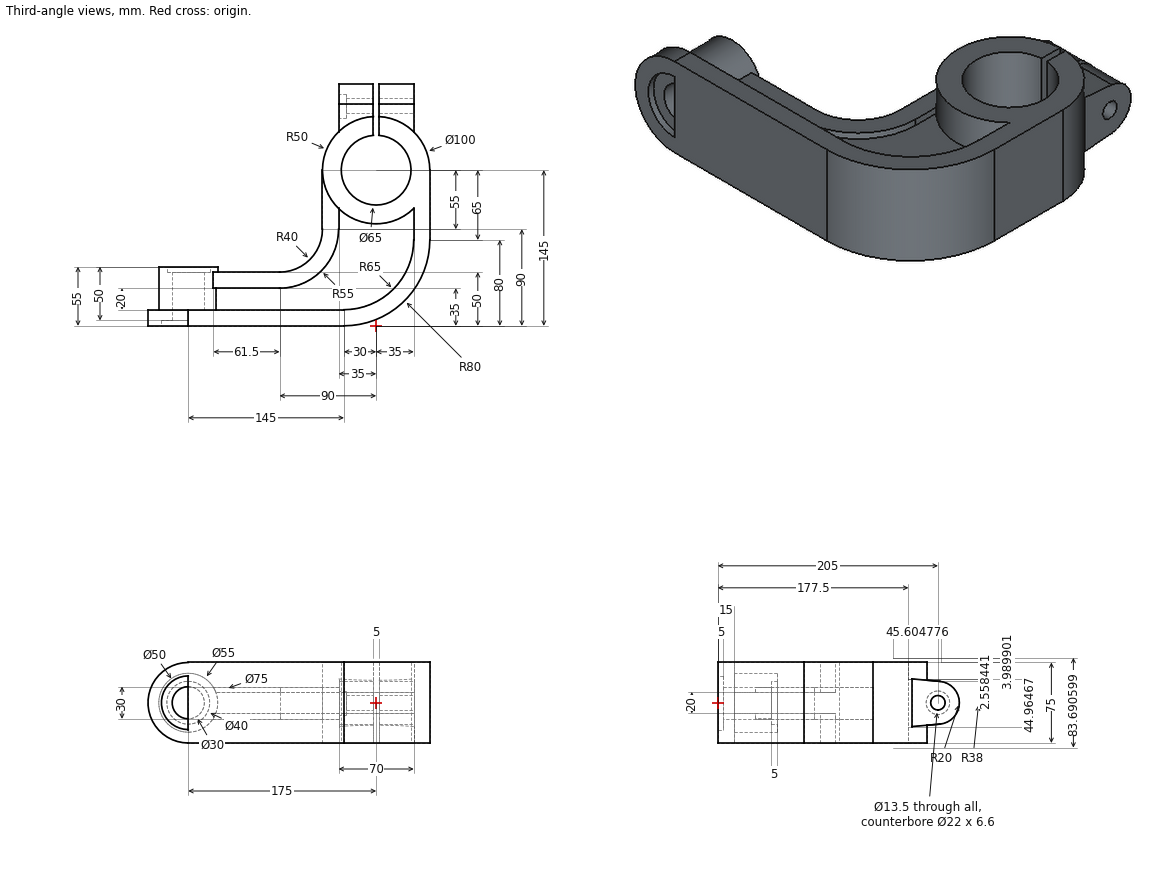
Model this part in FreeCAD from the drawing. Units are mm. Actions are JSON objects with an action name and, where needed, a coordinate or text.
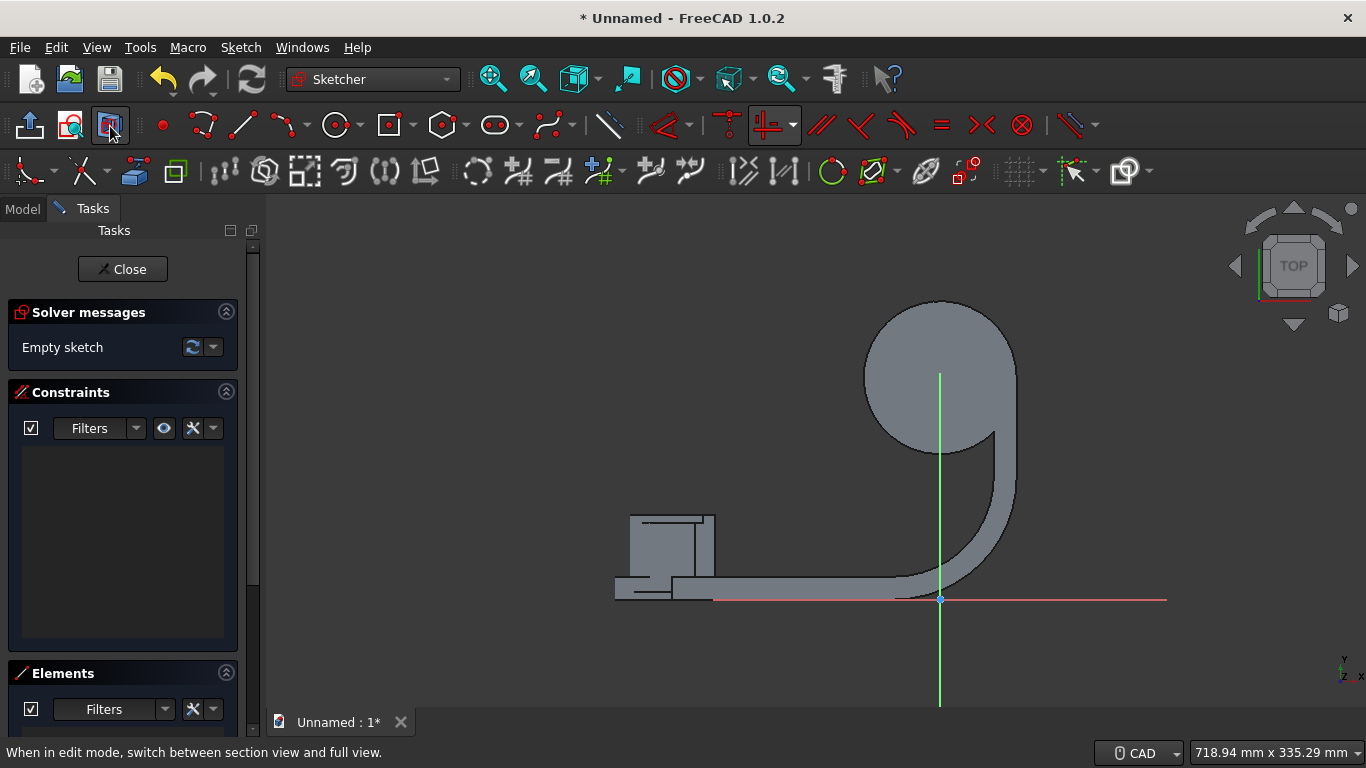
{"action": "scroll", "coordinate": [1023, 346], "scroll_direction": "up", "scroll_amount": 6}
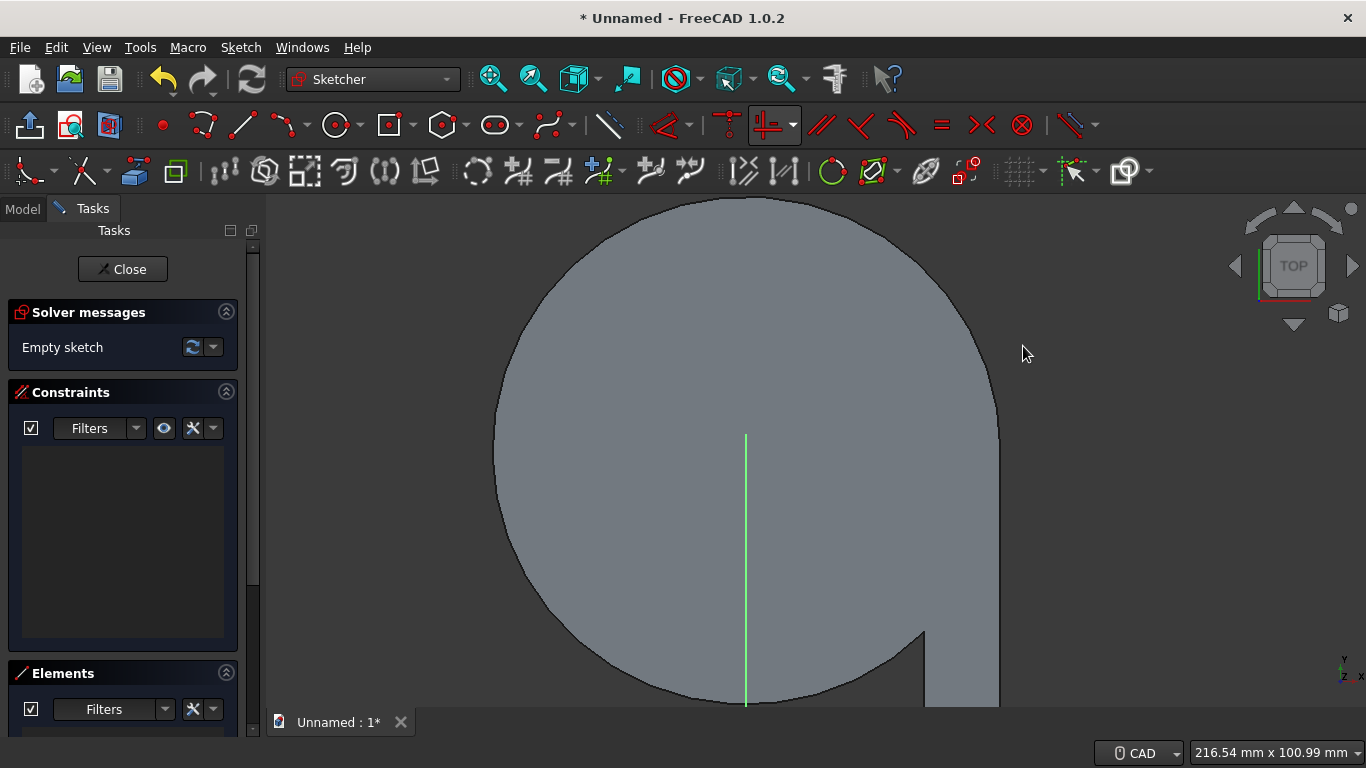
{"action": "key", "text": "g c"}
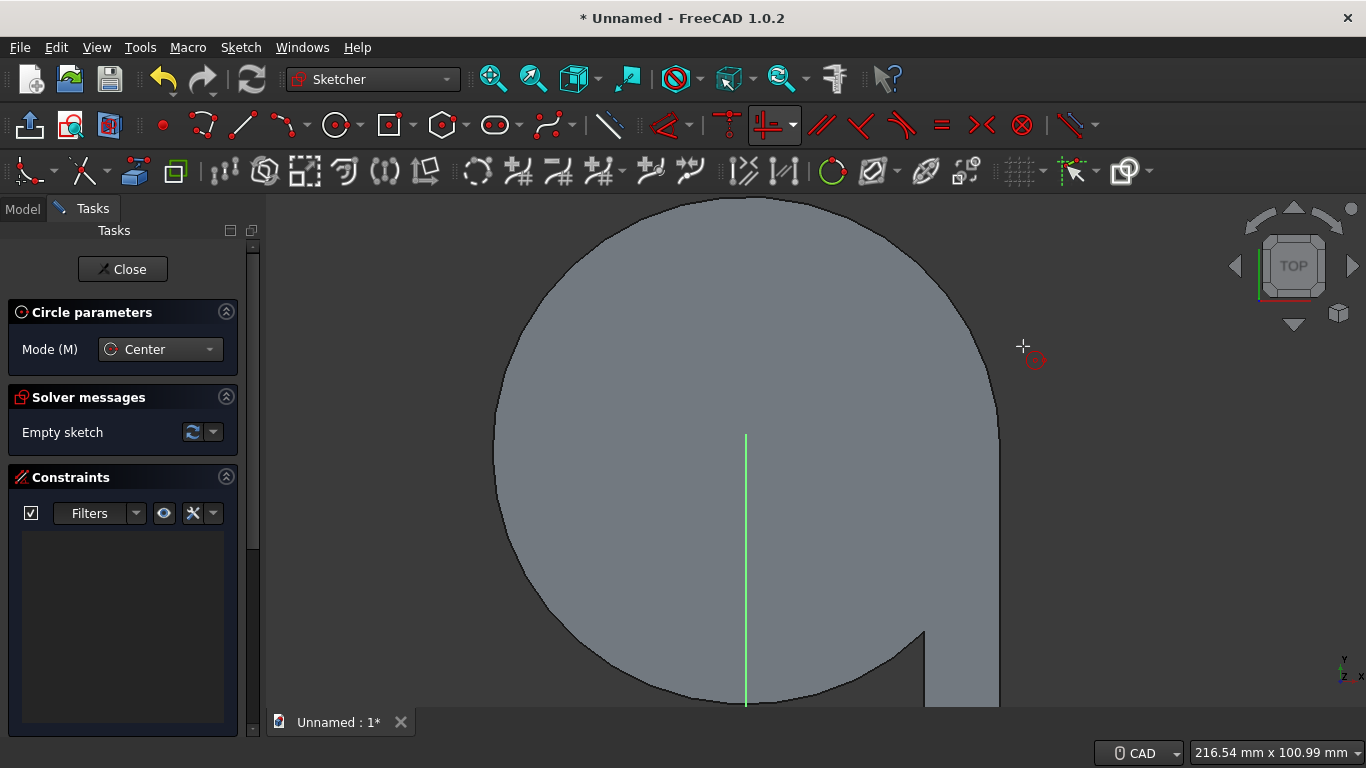
{"action": "left_click", "coordinate": [746, 451]}
{"action": "left_click", "coordinate": [863, 334]}
{"action": "key", "text": "Escape"}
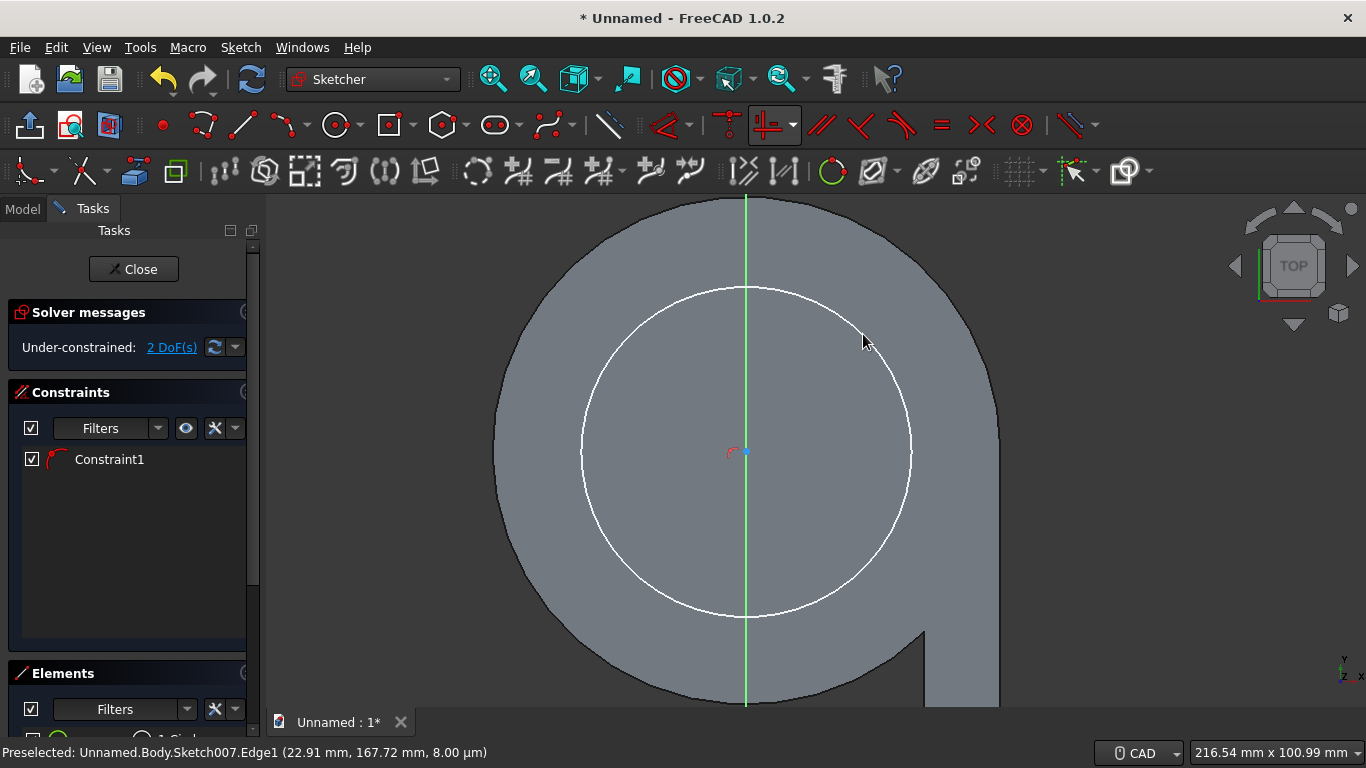
{"action": "key", "text": "d"}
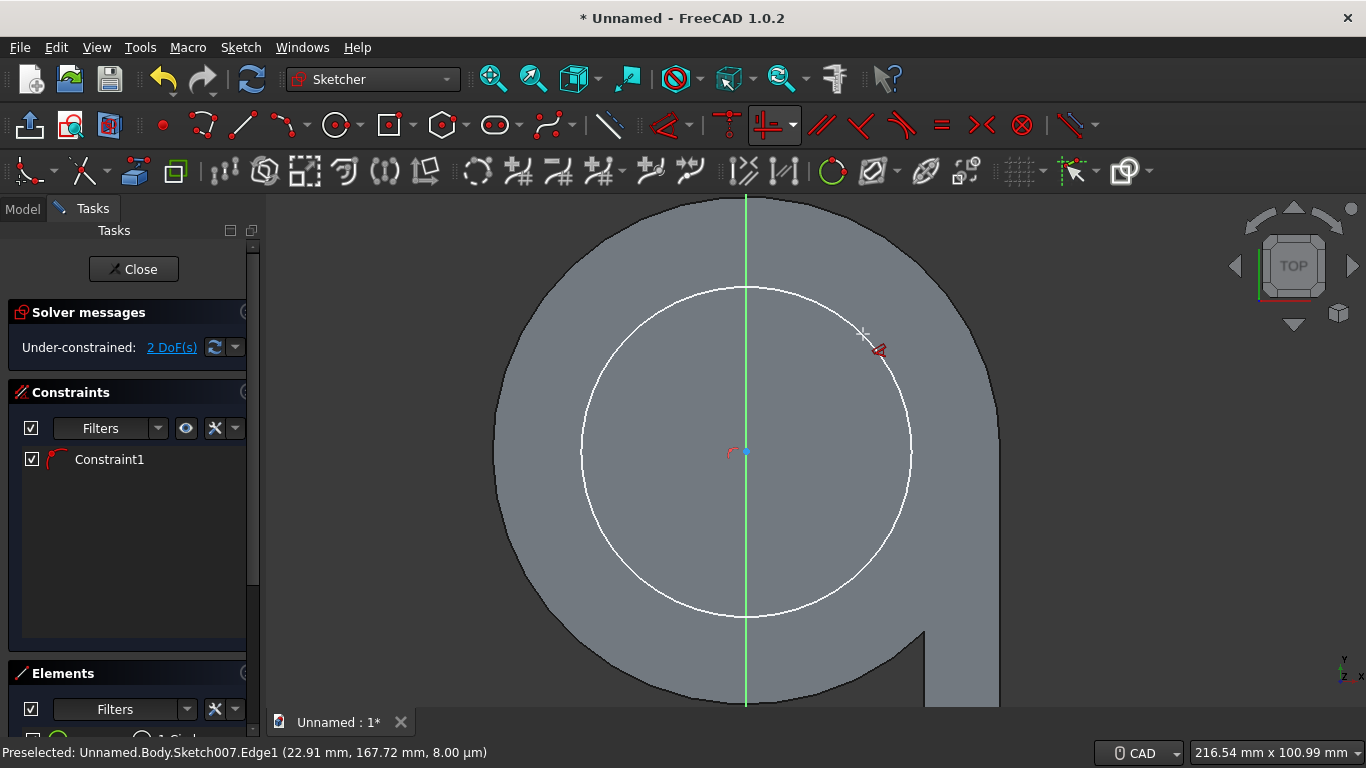
{"action": "left_click", "coordinate": [863, 335]}
{"action": "left_click", "coordinate": [886, 312]}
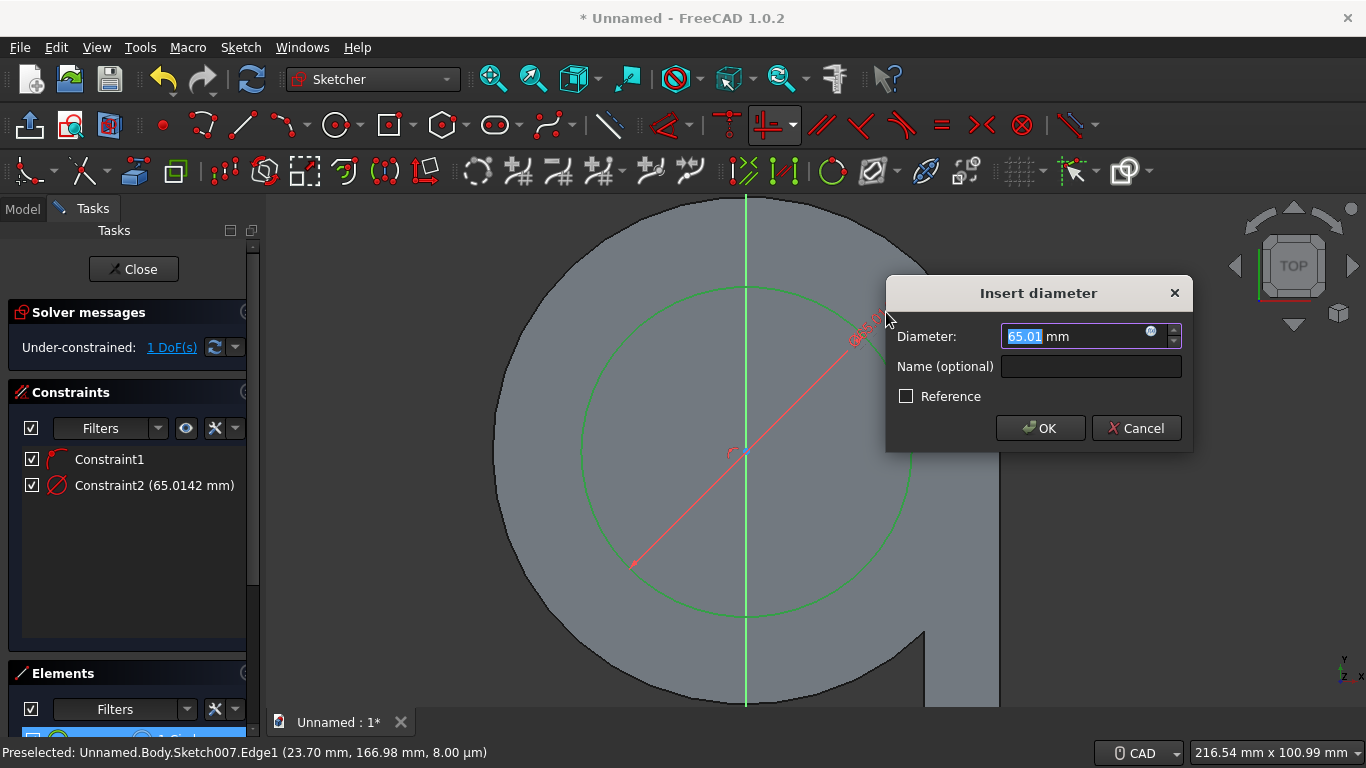
{"action": "type", "text": "65"}
{"action": "key", "text": "Return"}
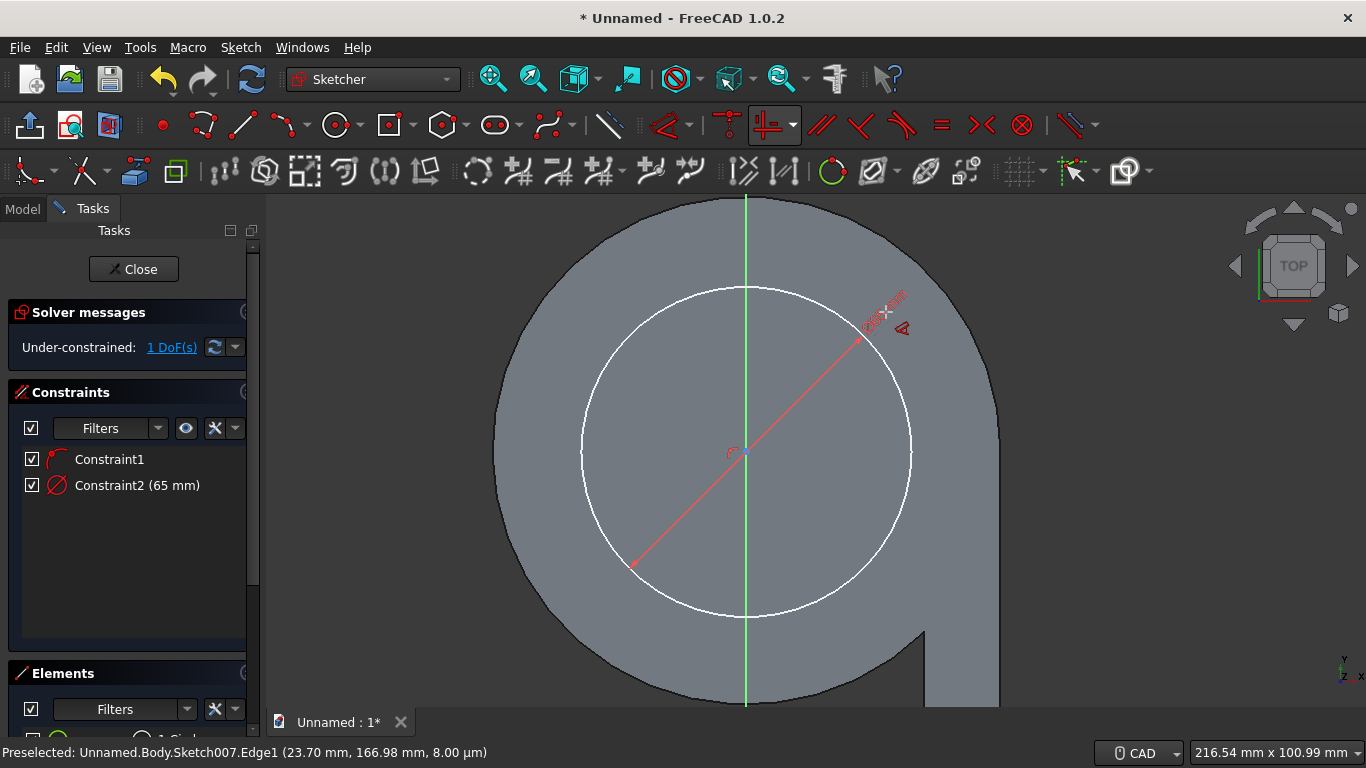
{"action": "left_click", "coordinate": [746, 452]}
{"action": "left_click", "coordinate": [780, 566]}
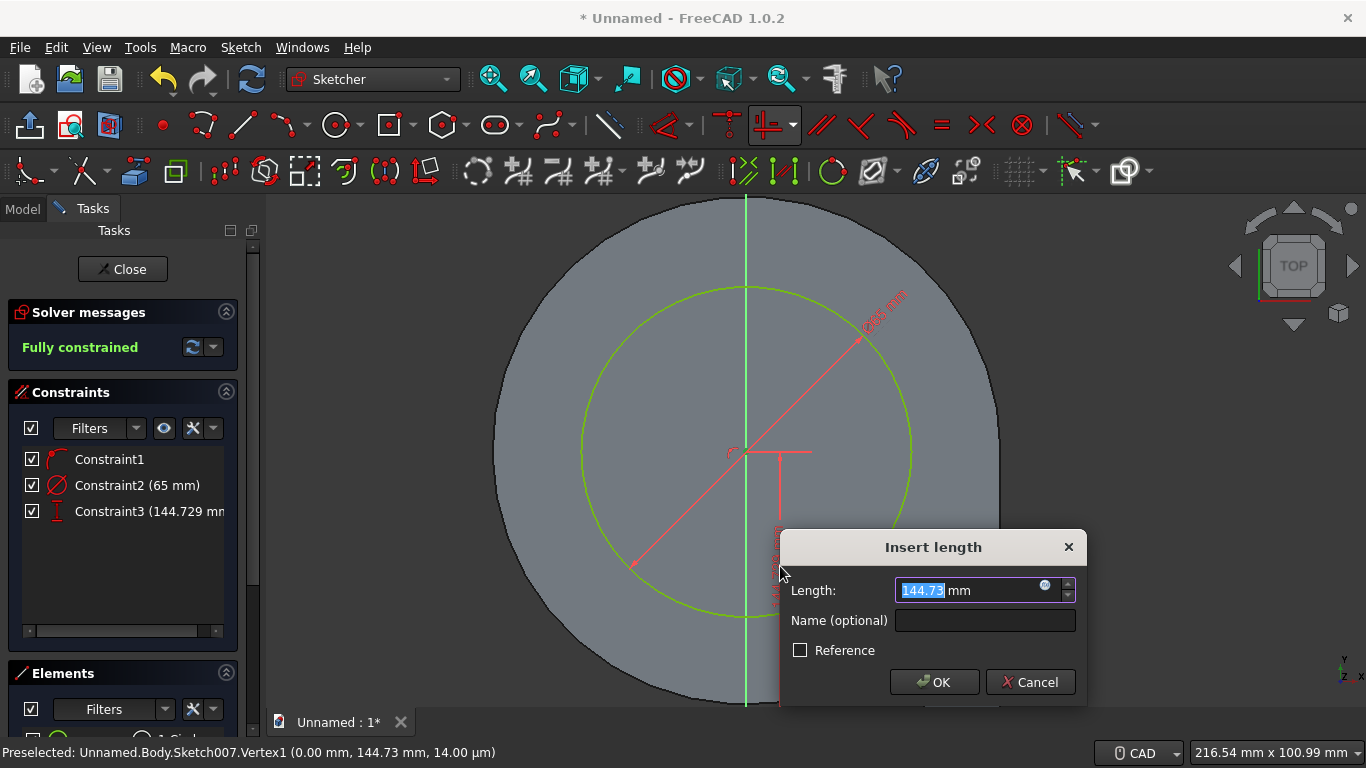
{"action": "type", "text": "145"}
{"action": "key", "text": "Return"}
{"action": "key", "text": "Escape"}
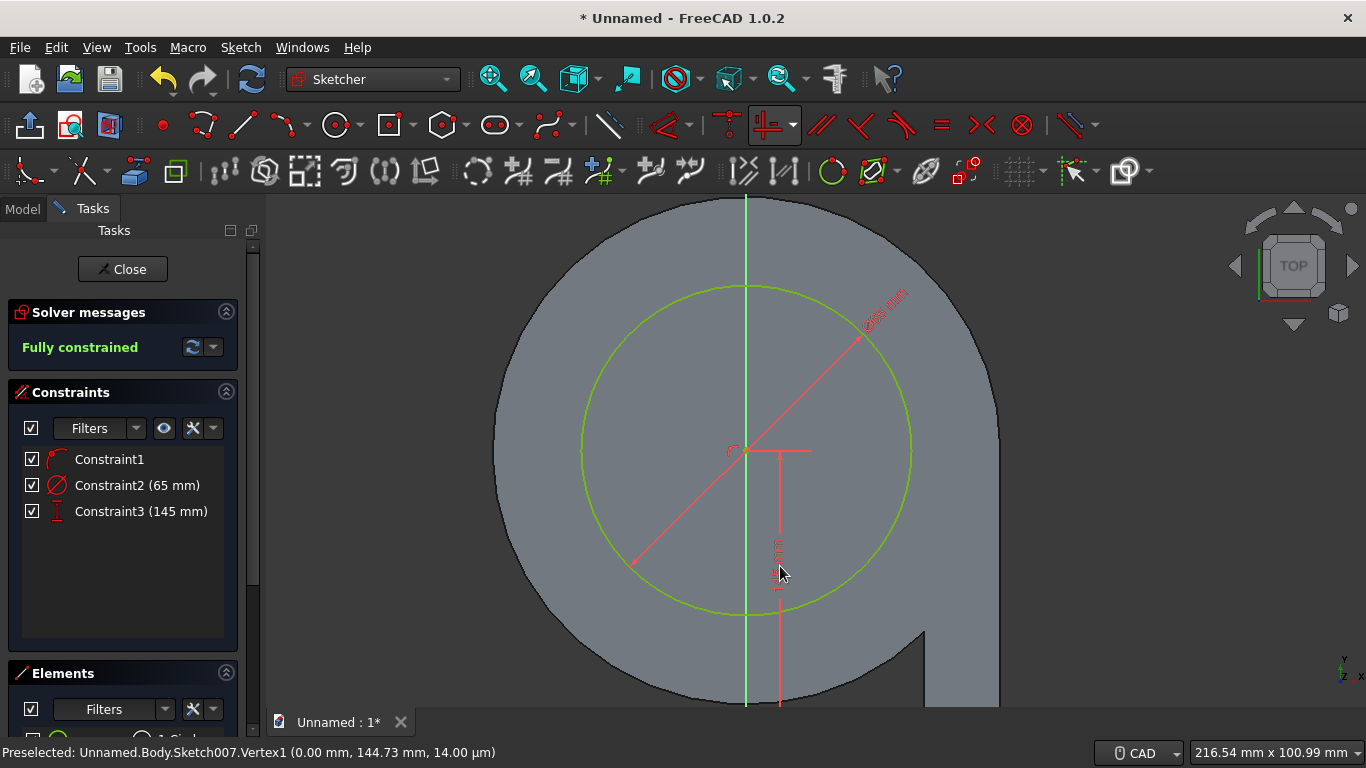
{"action": "left_click", "coordinate": [123, 269]}